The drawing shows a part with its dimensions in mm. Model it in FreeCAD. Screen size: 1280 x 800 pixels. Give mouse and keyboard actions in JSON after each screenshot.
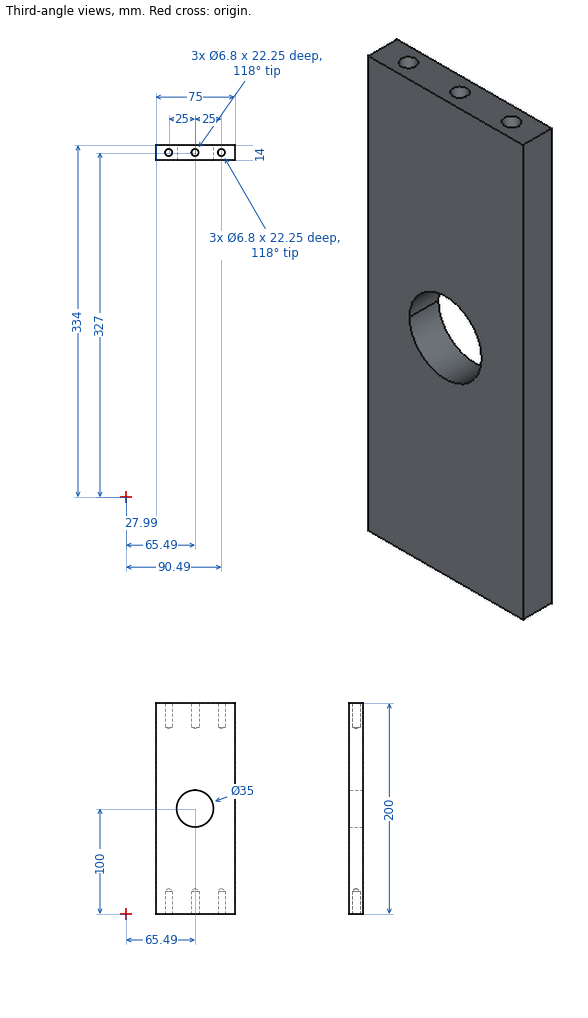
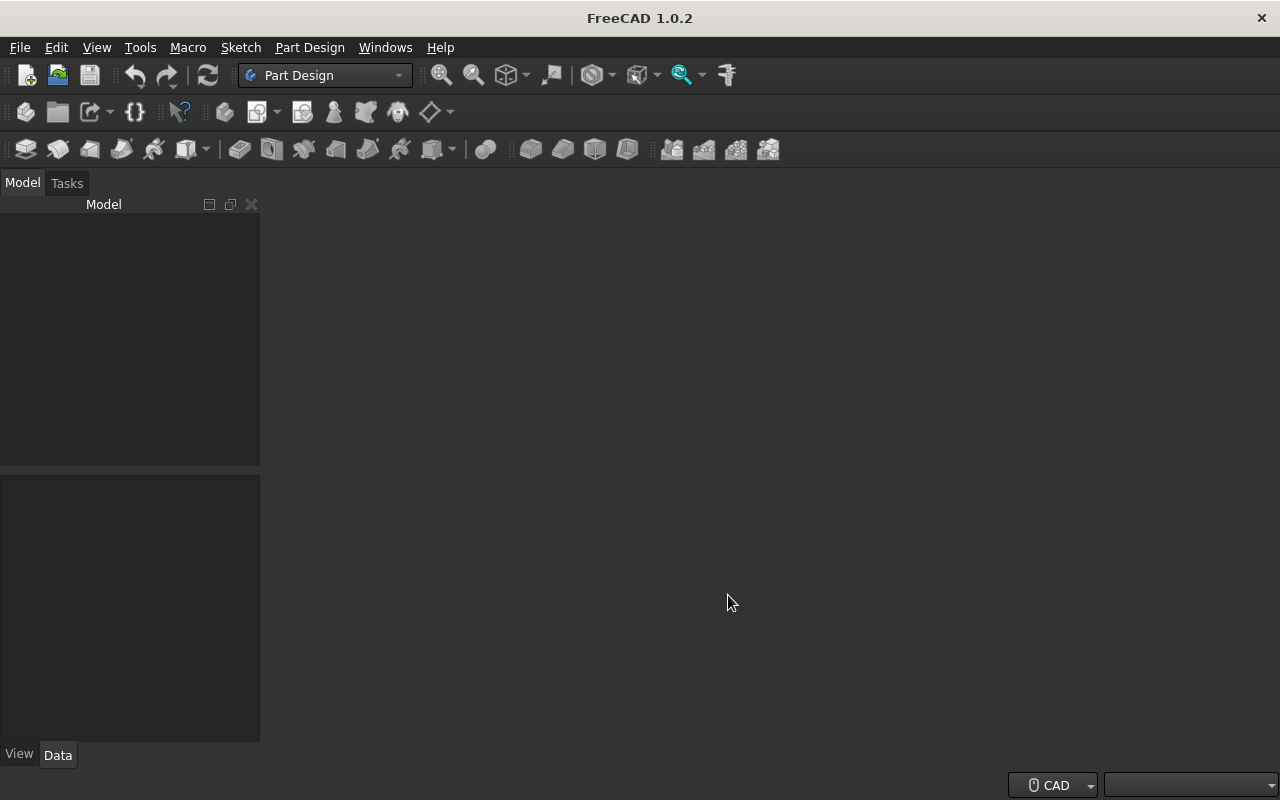
{"action": "key", "text": "ctrl+n"}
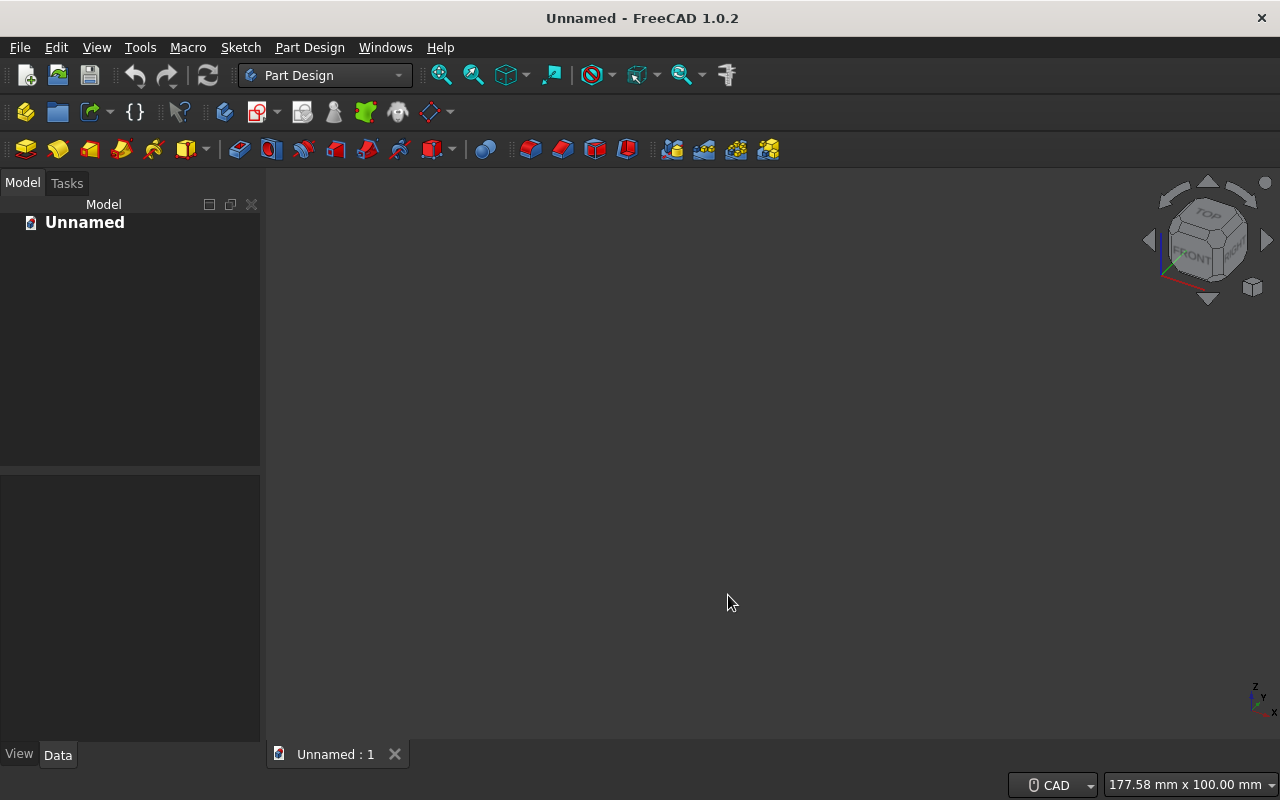
{"action": "left_click", "coordinate": [258, 112]}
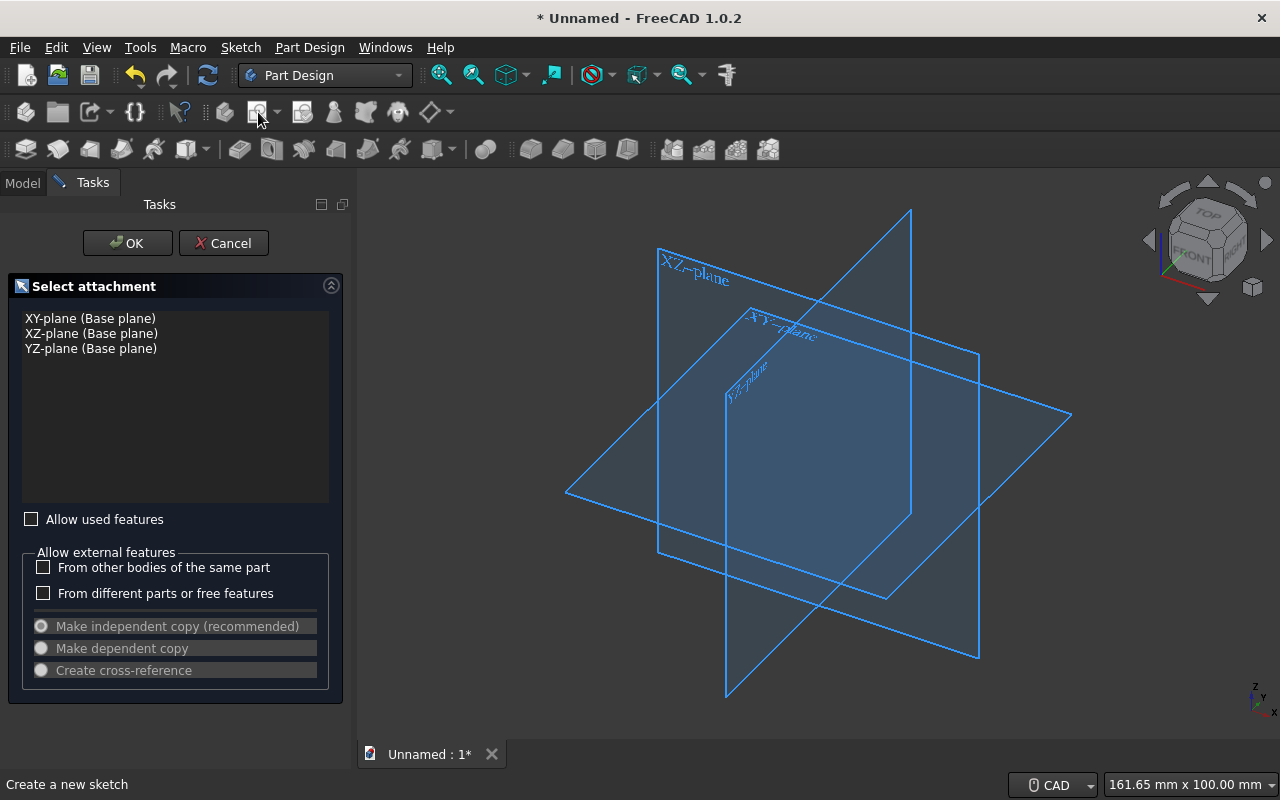
{"action": "left_click", "coordinate": [82, 318]}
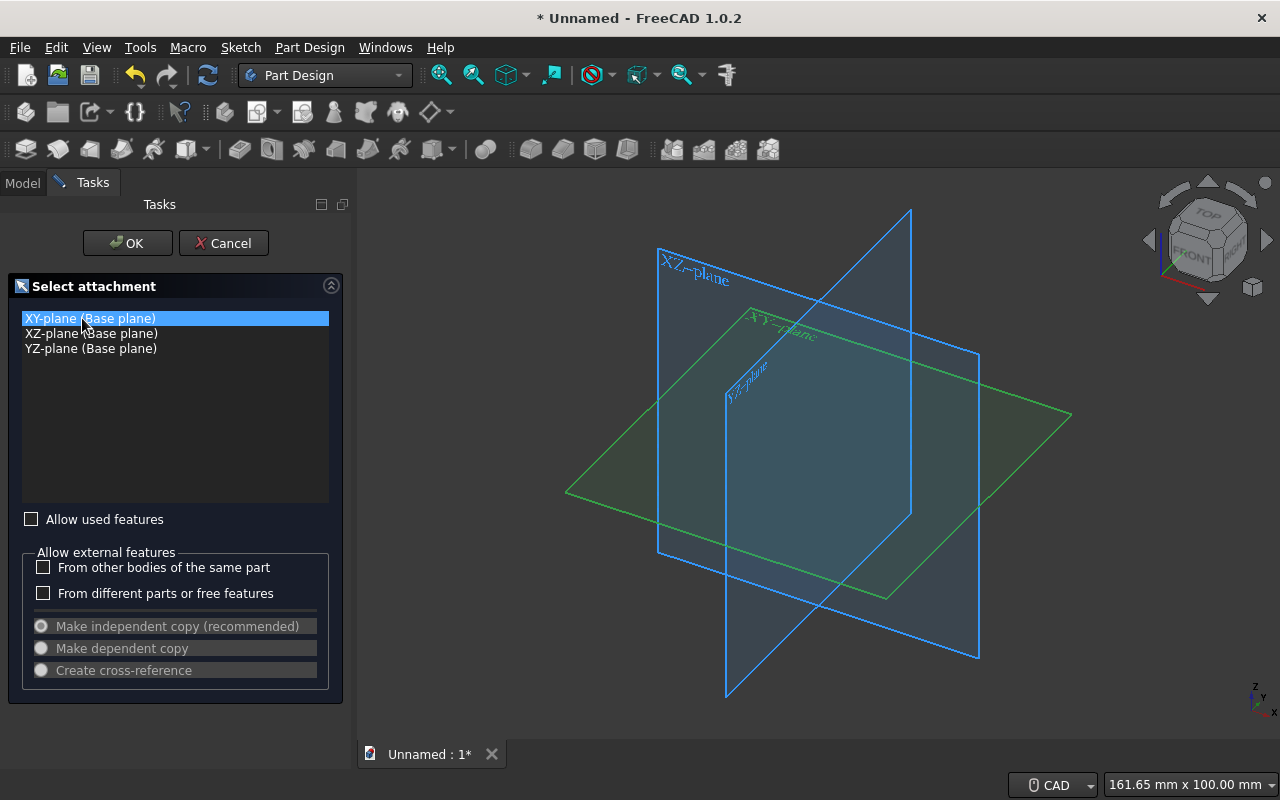
{"action": "left_click", "coordinate": [128, 243]}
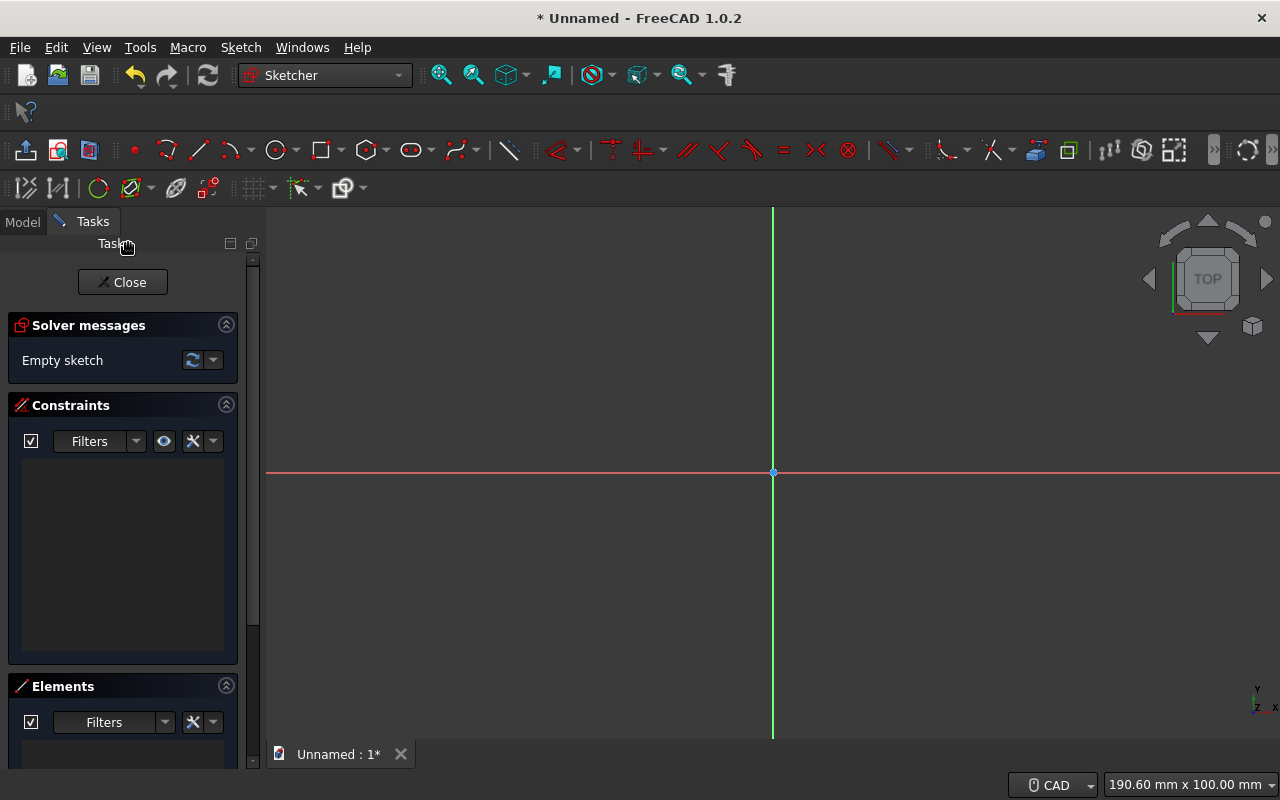
{"action": "scroll", "coordinate": [704, 473], "scroll_direction": "down", "scroll_amount": 5}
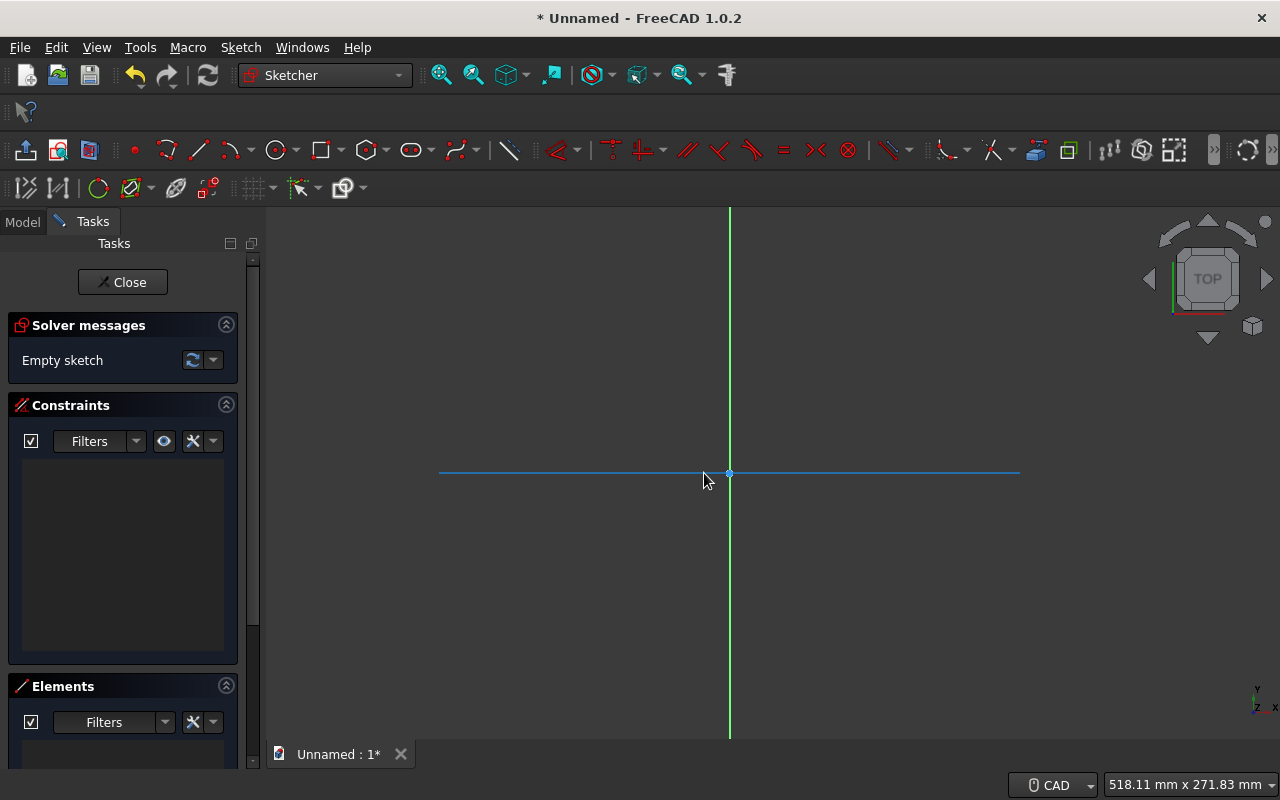
{"action": "scroll", "coordinate": [704, 473], "scroll_direction": "down", "scroll_amount": 5}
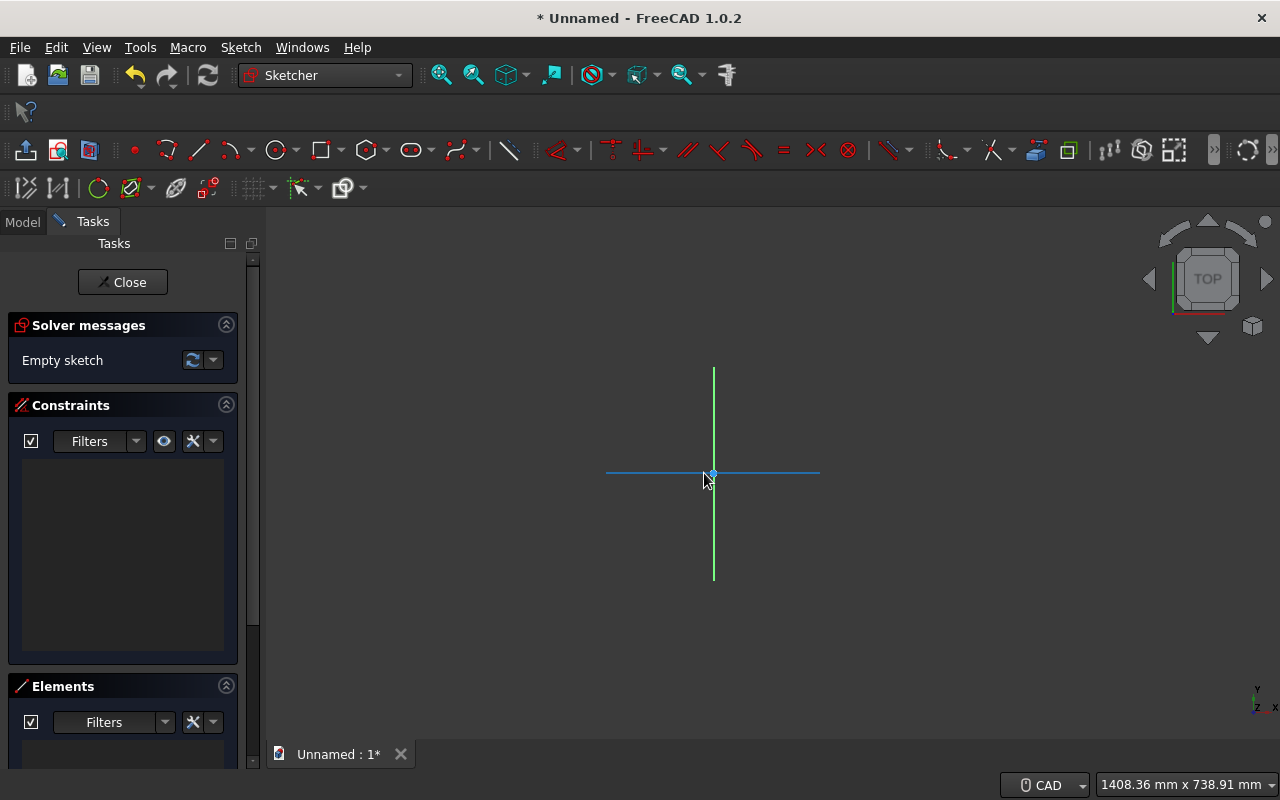
{"action": "scroll", "coordinate": [704, 473], "scroll_direction": "down", "scroll_amount": 5}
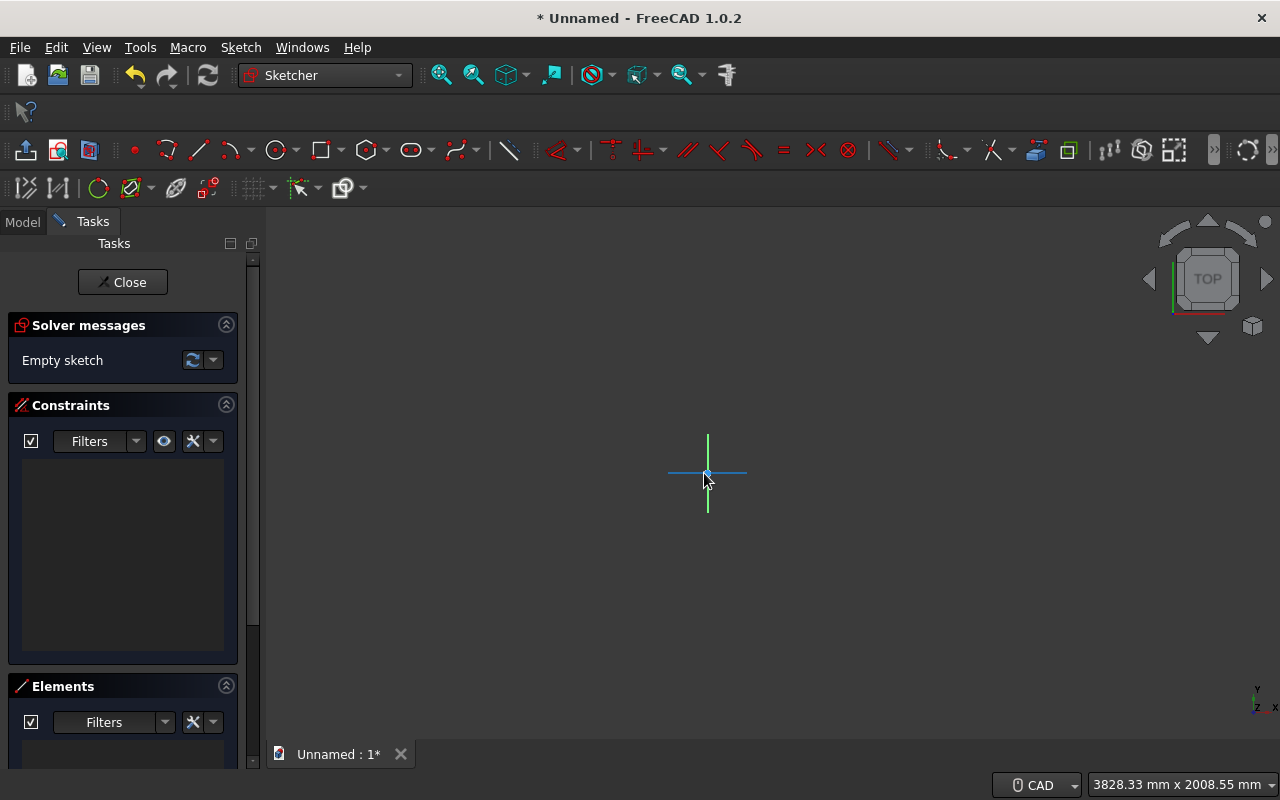
{"action": "scroll", "coordinate": [726, 382], "scroll_direction": "up", "scroll_amount": 15}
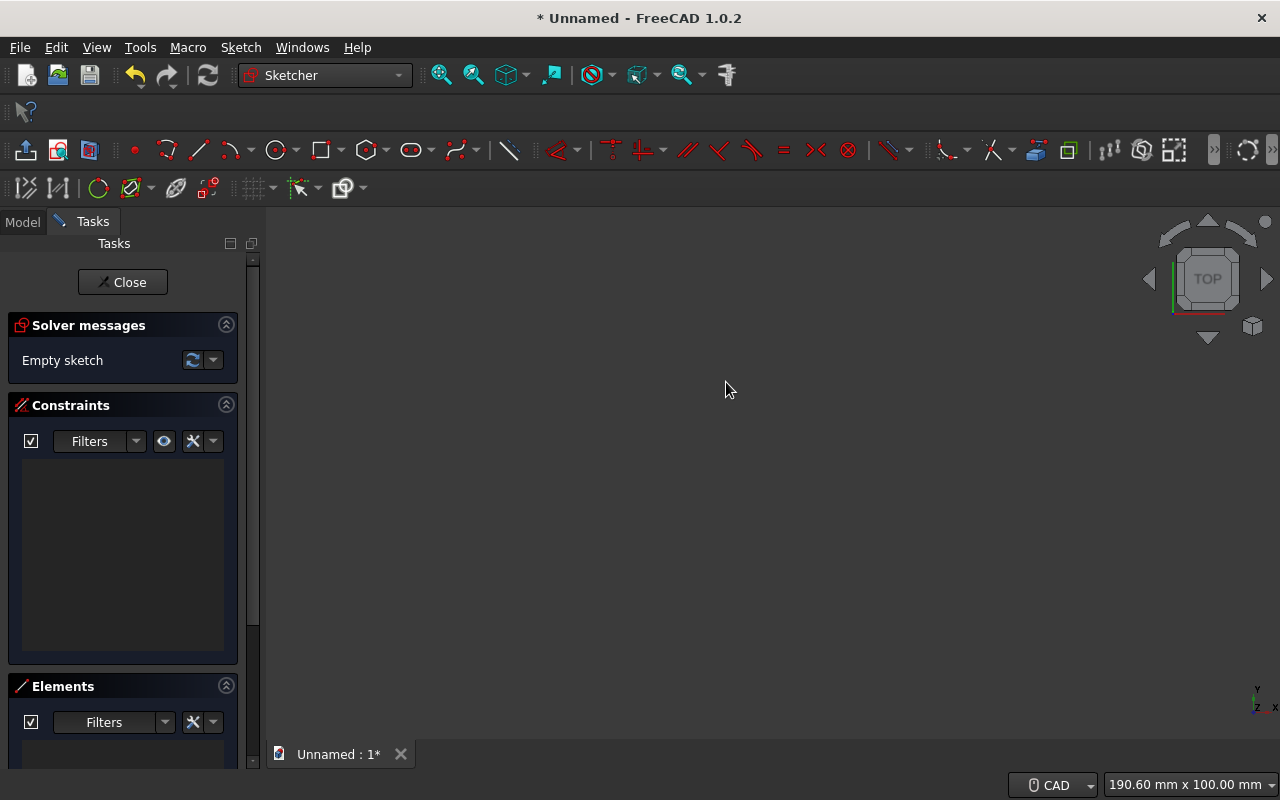
{"action": "scroll", "coordinate": [694, 474], "scroll_direction": "up", "scroll_amount": 2}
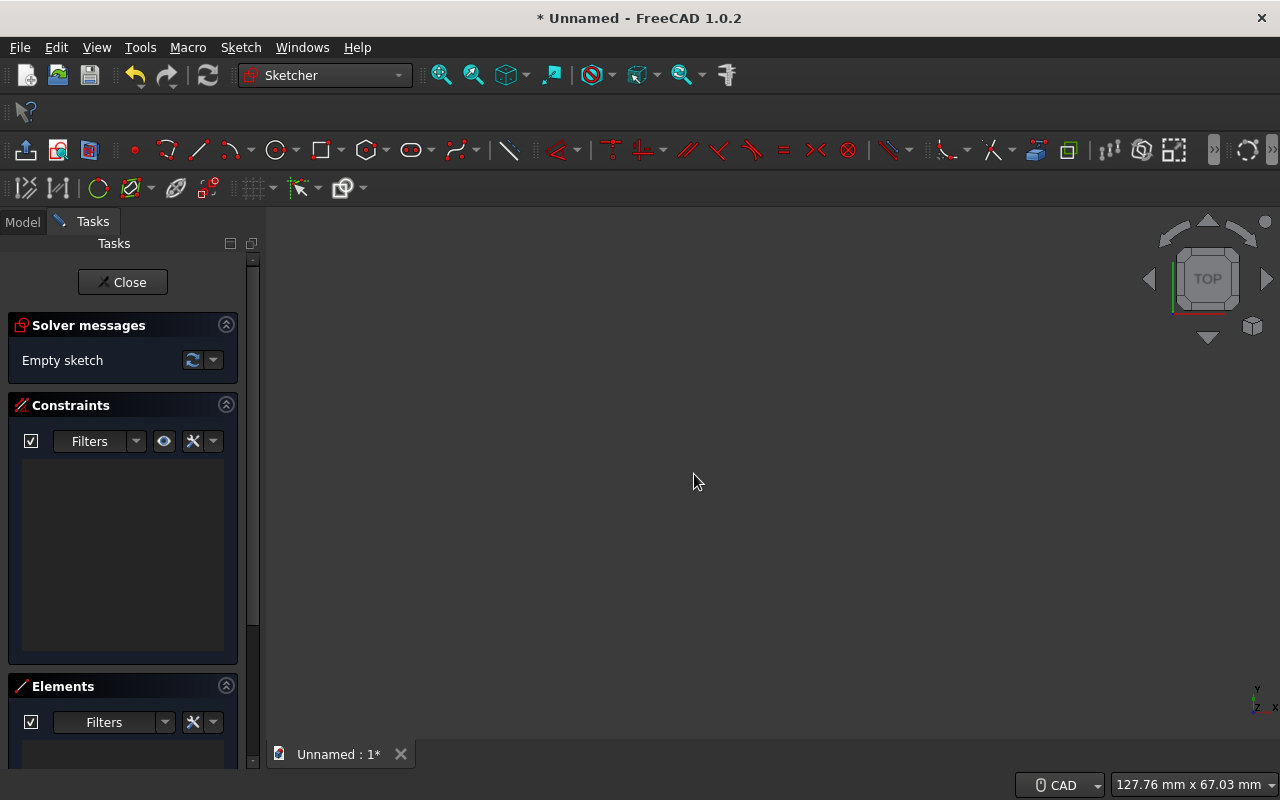
{"action": "left_click", "coordinate": [322, 150]}